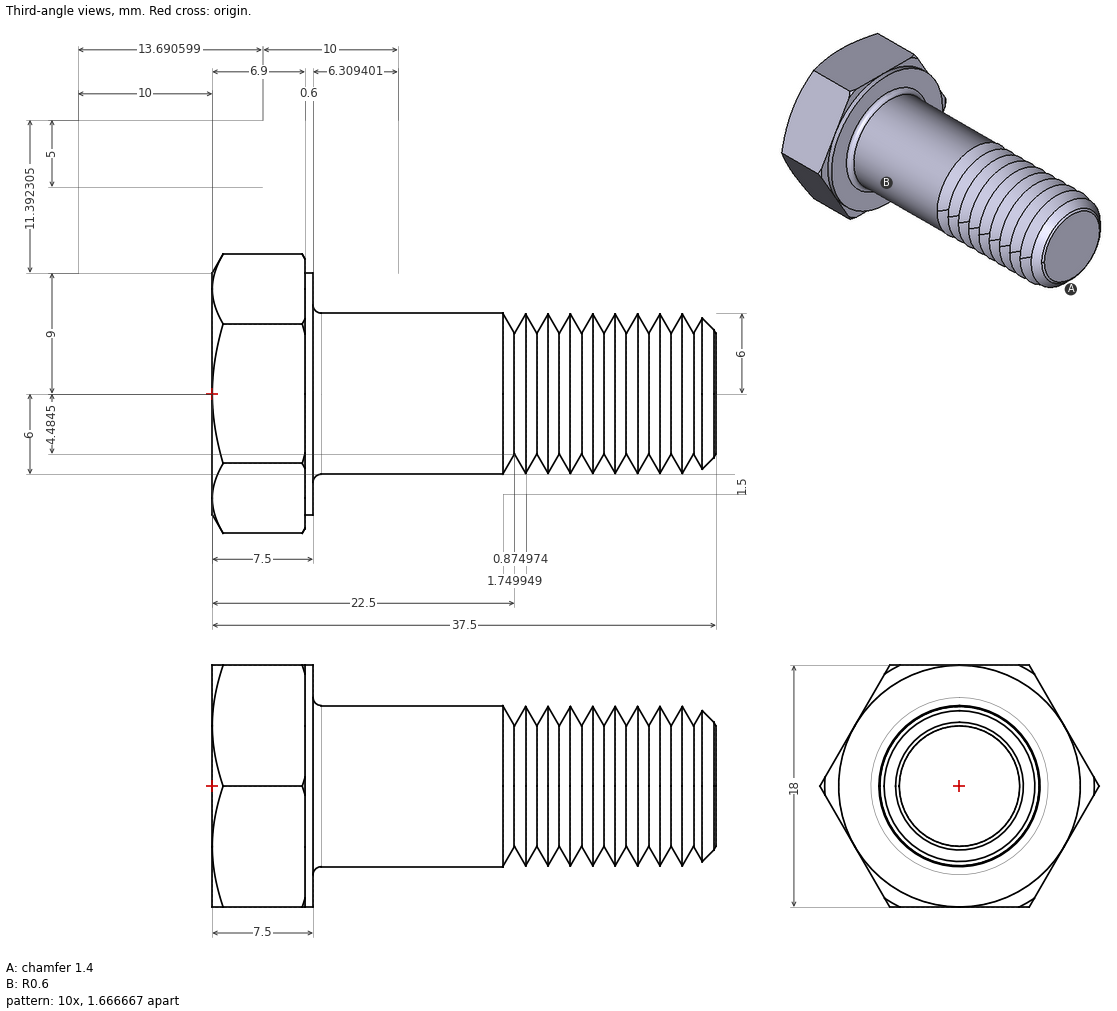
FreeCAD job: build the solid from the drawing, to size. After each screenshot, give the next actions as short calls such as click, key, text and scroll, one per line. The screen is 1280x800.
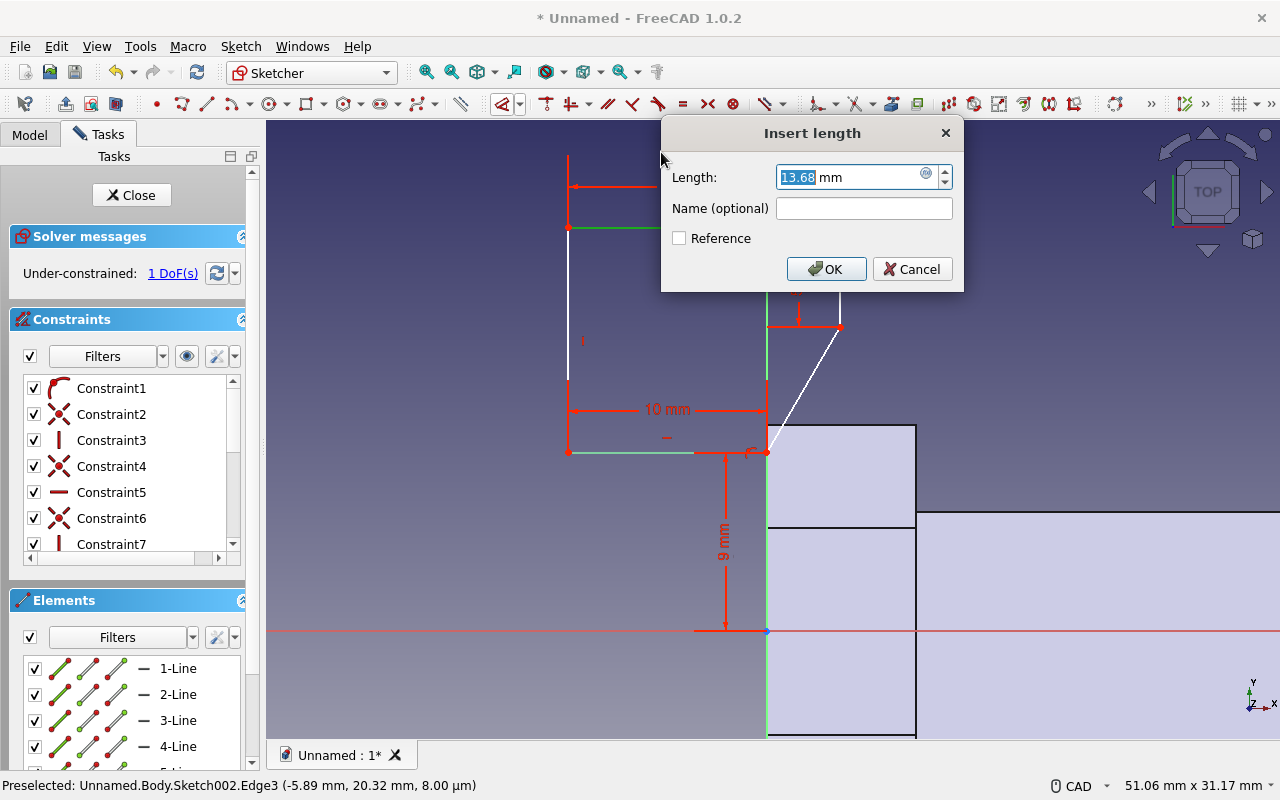
text(13.690599)
key(Return)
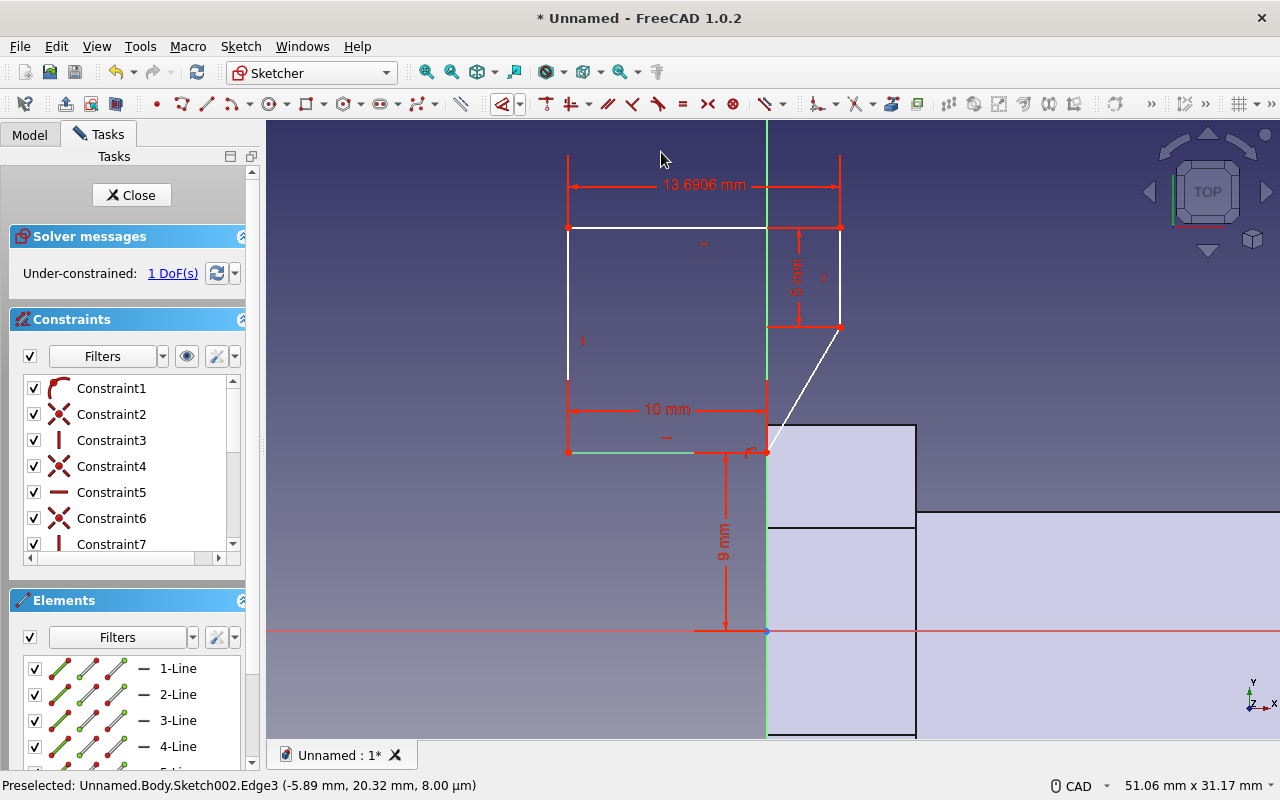
click(568, 295)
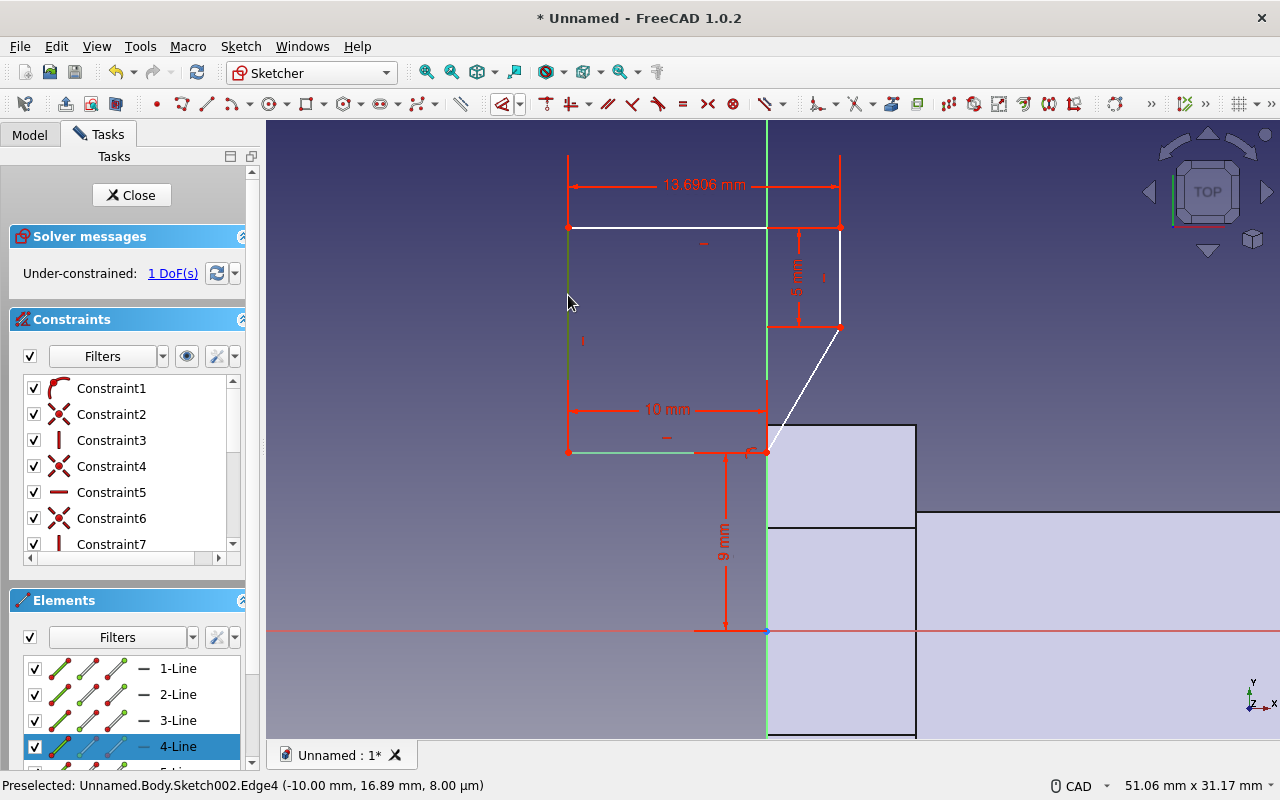
click(520, 104)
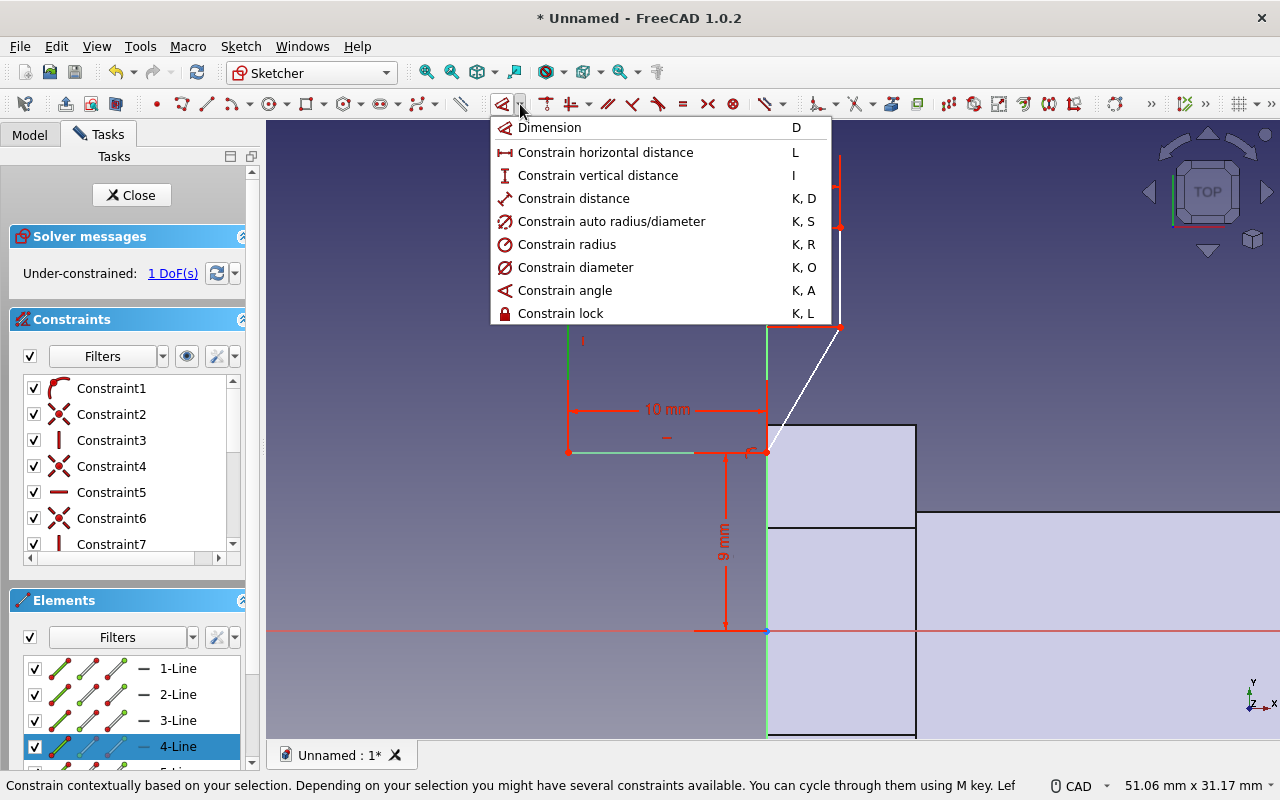
click(661, 176)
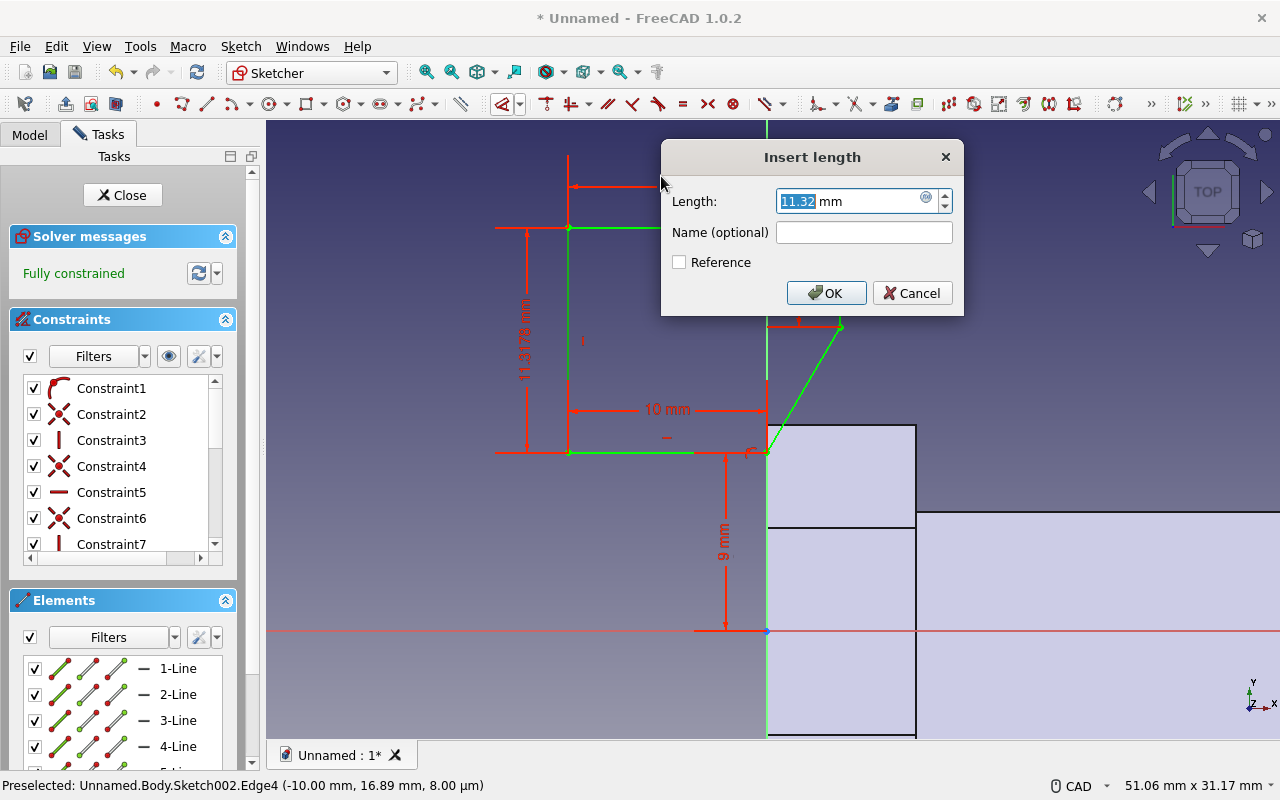
text(11.392305)
key(Return)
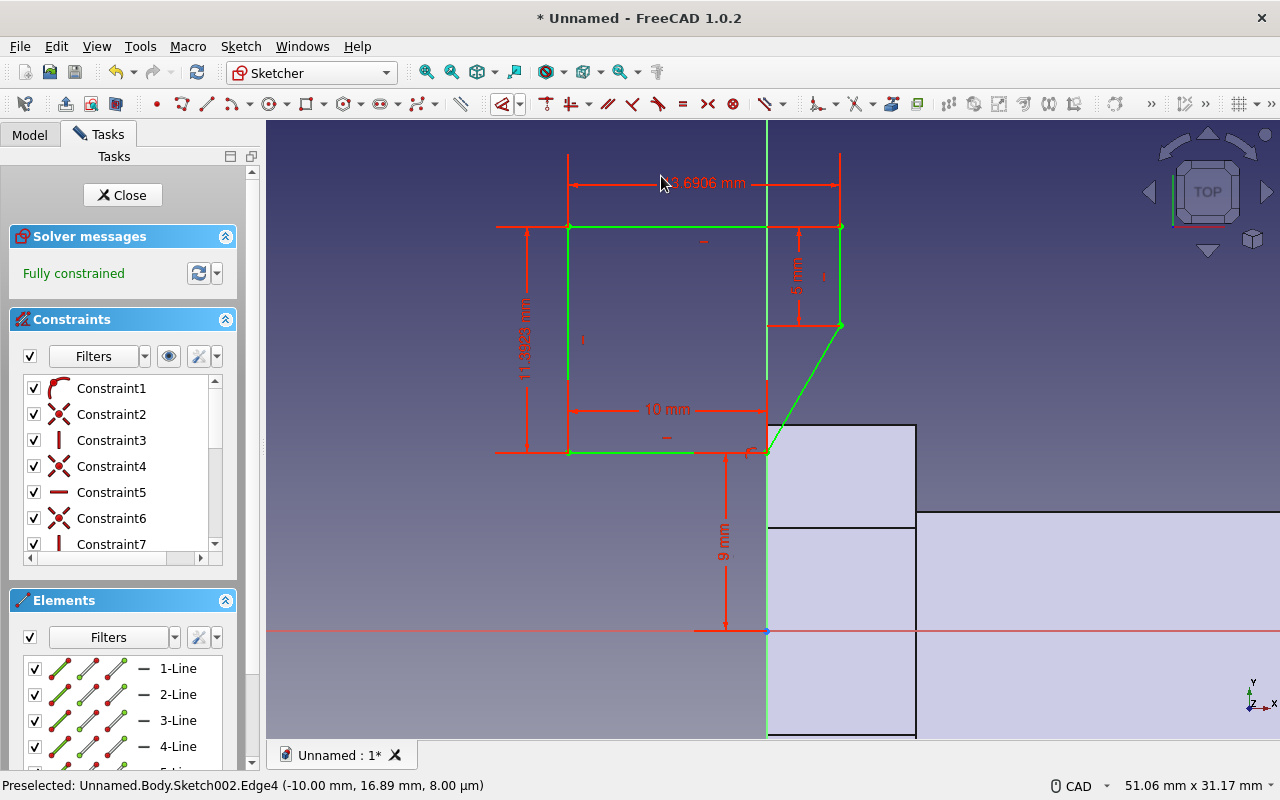
click(123, 195)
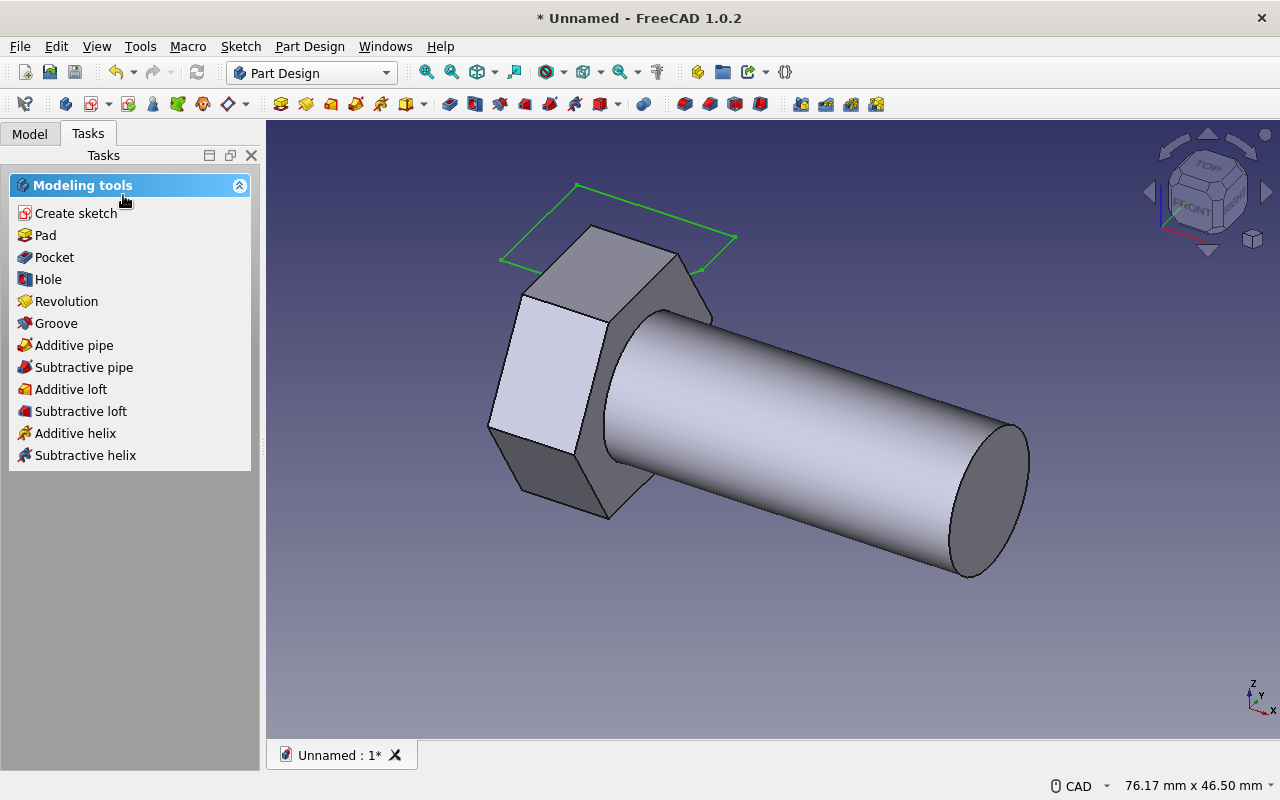
click(500, 104)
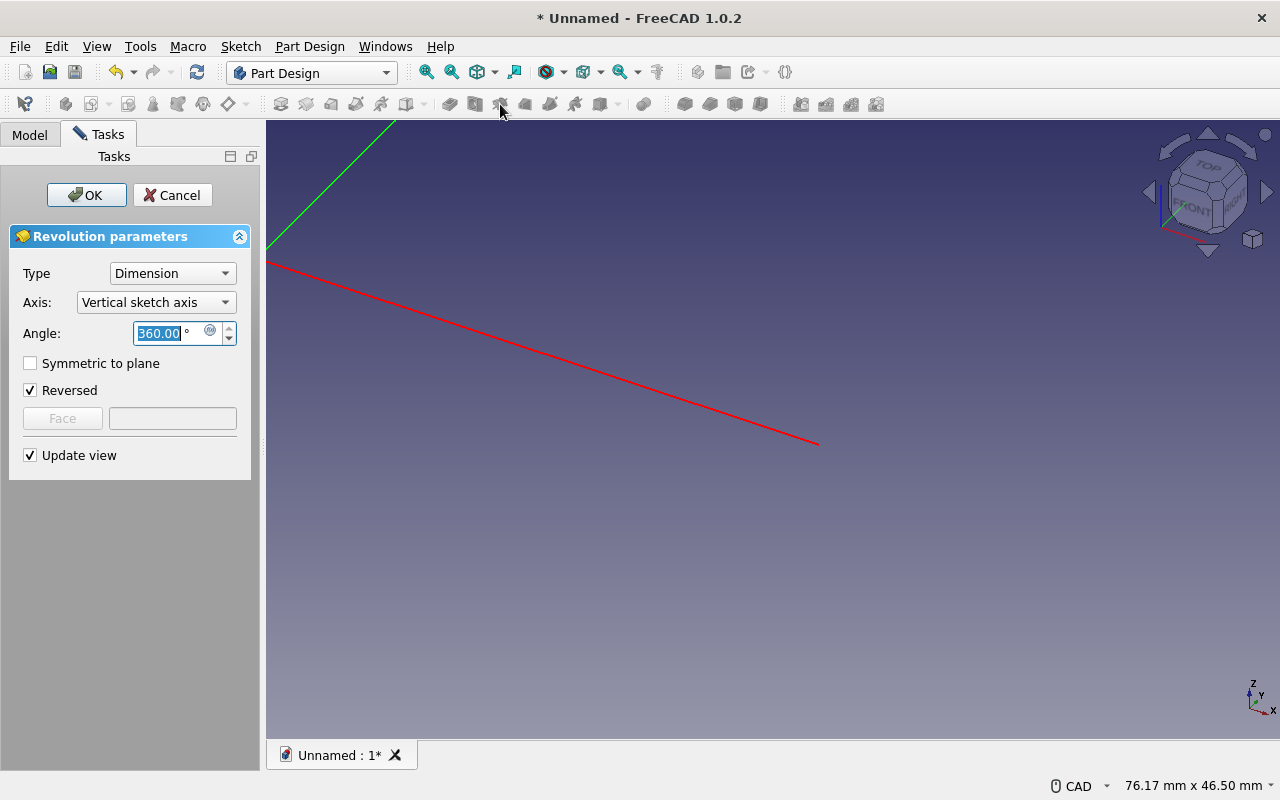
click(157, 302)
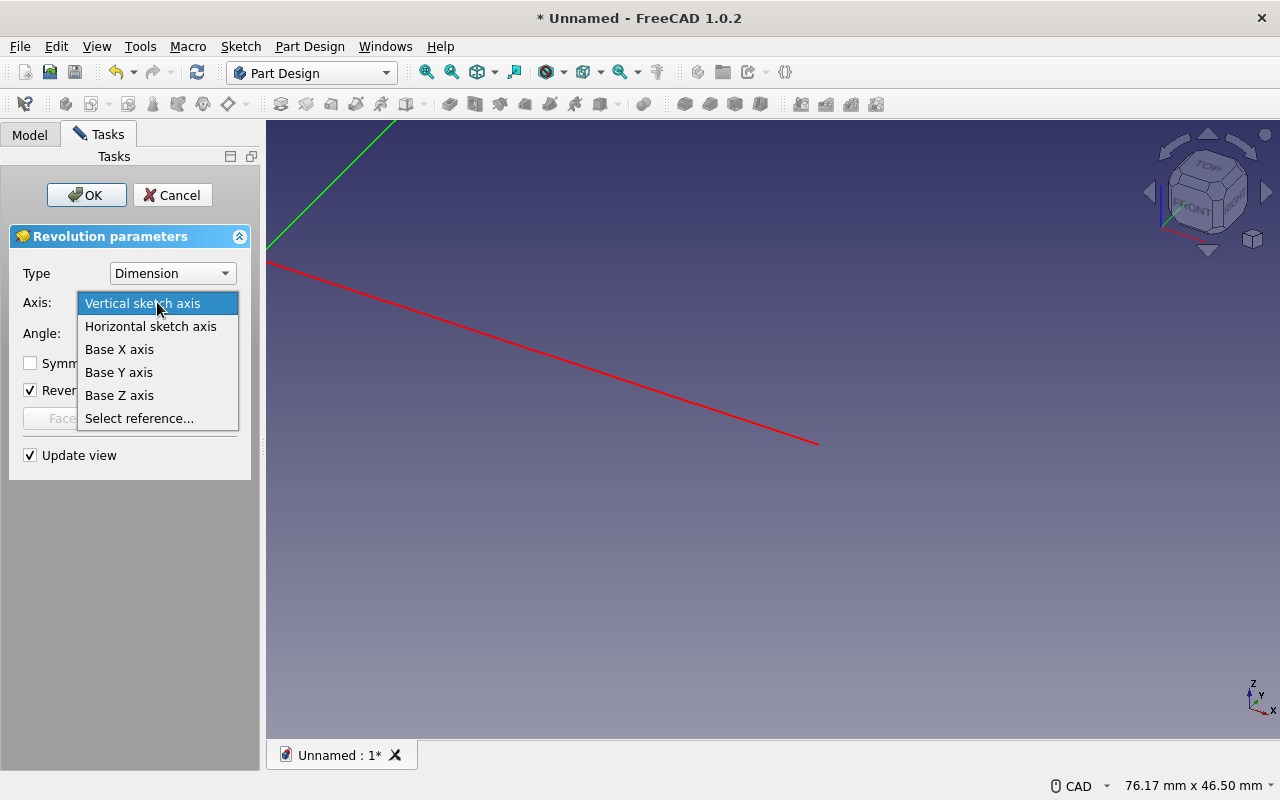
click(156, 326)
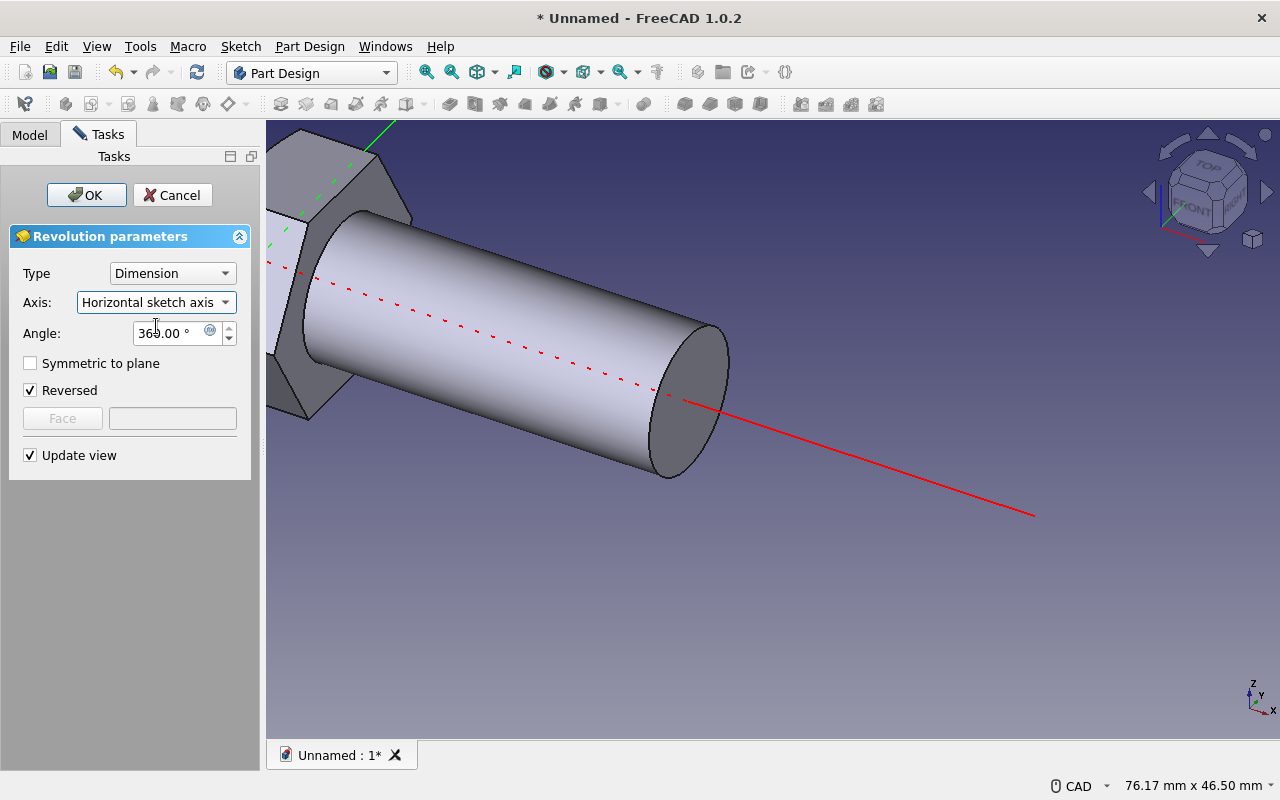
click(87, 195)